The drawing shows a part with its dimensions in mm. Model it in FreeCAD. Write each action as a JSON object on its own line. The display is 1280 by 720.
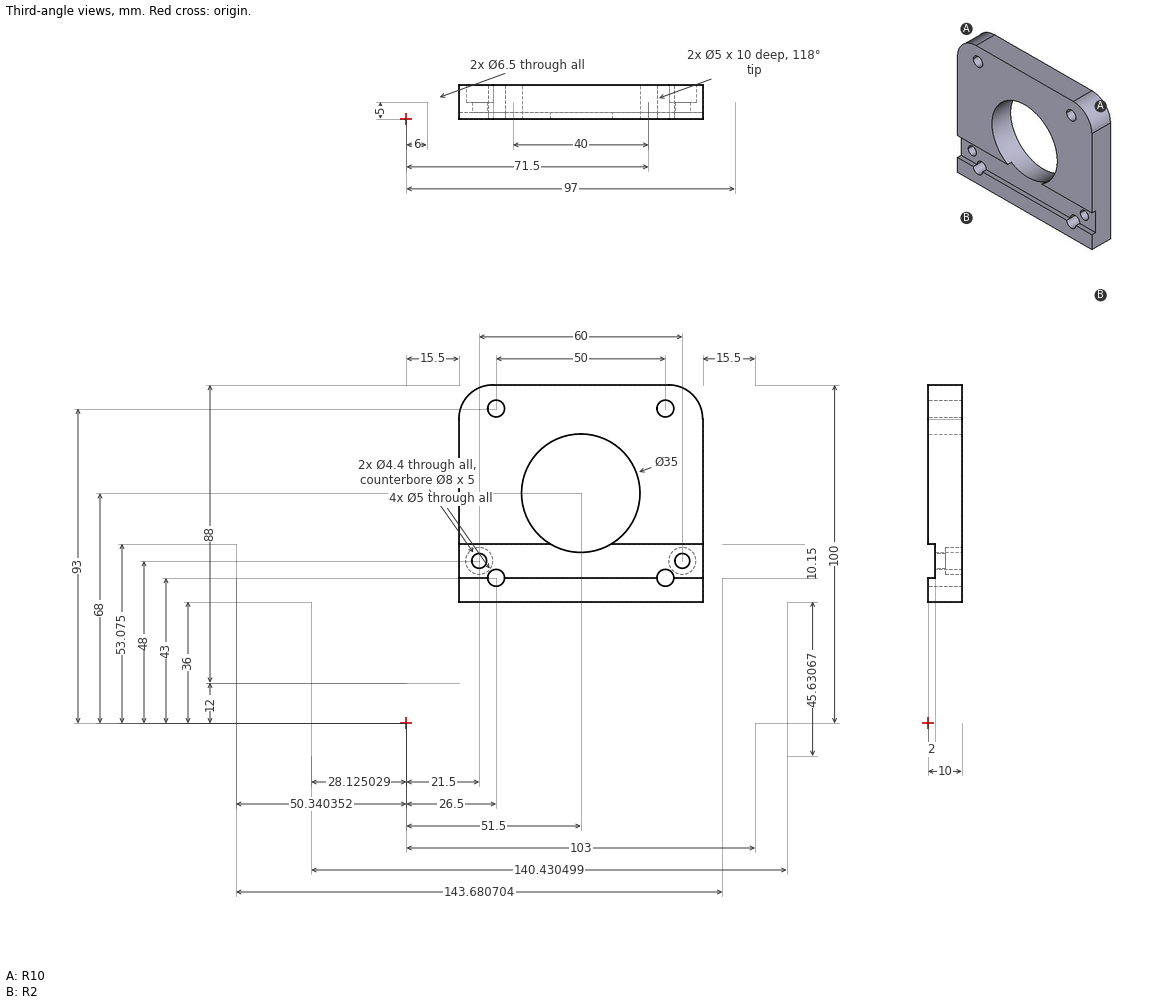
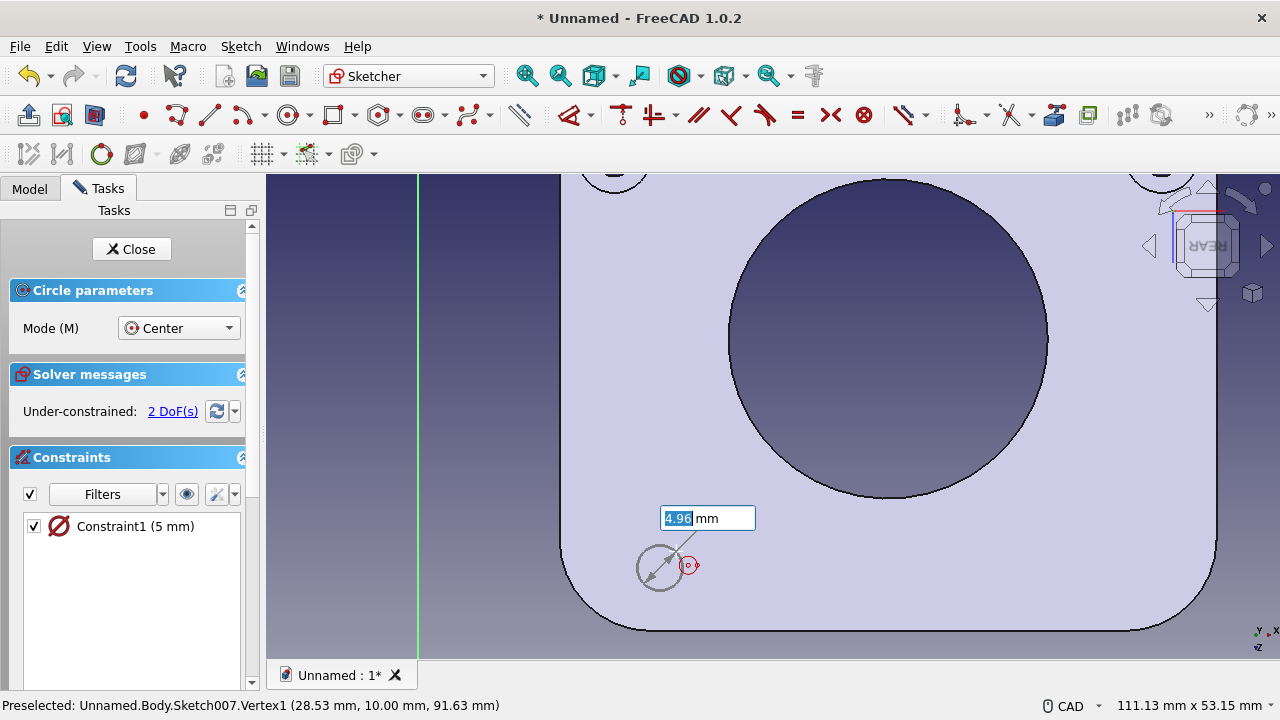
{"action": "type", "text": "5"}
{"action": "key", "text": "Return"}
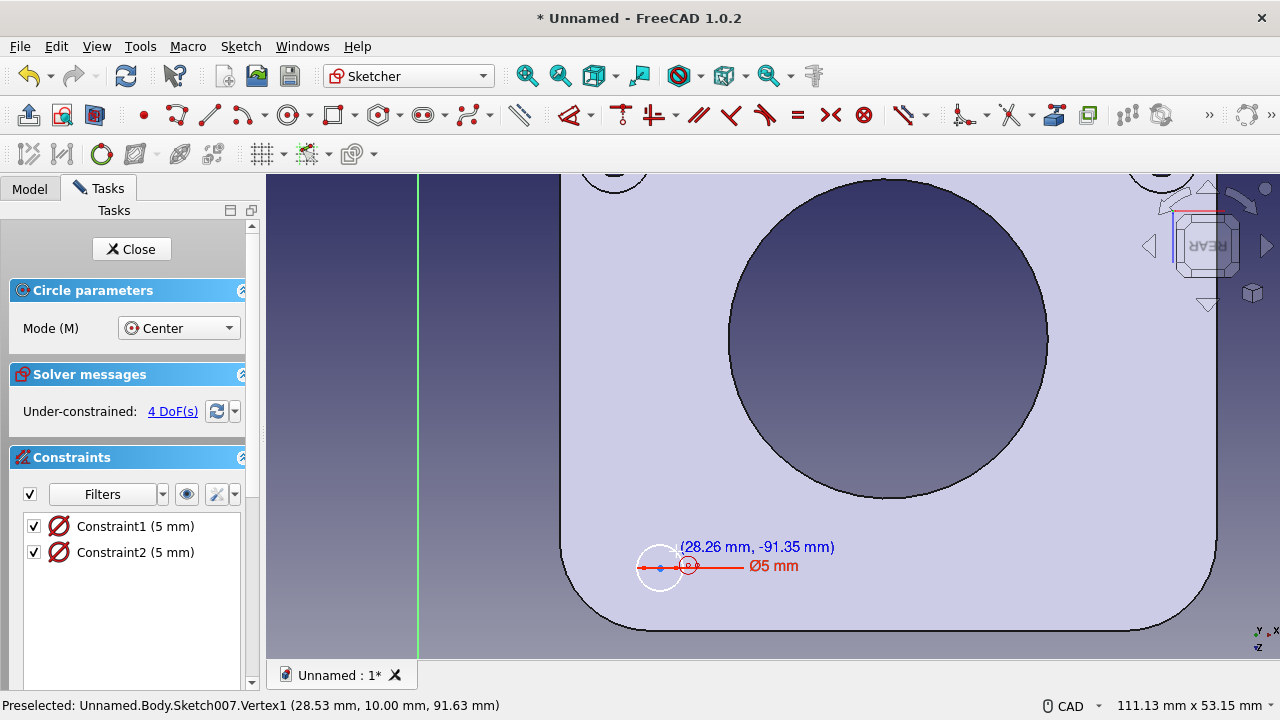
{"action": "scroll", "coordinate": [661, 569], "scroll_direction": "down", "scroll_amount": 5}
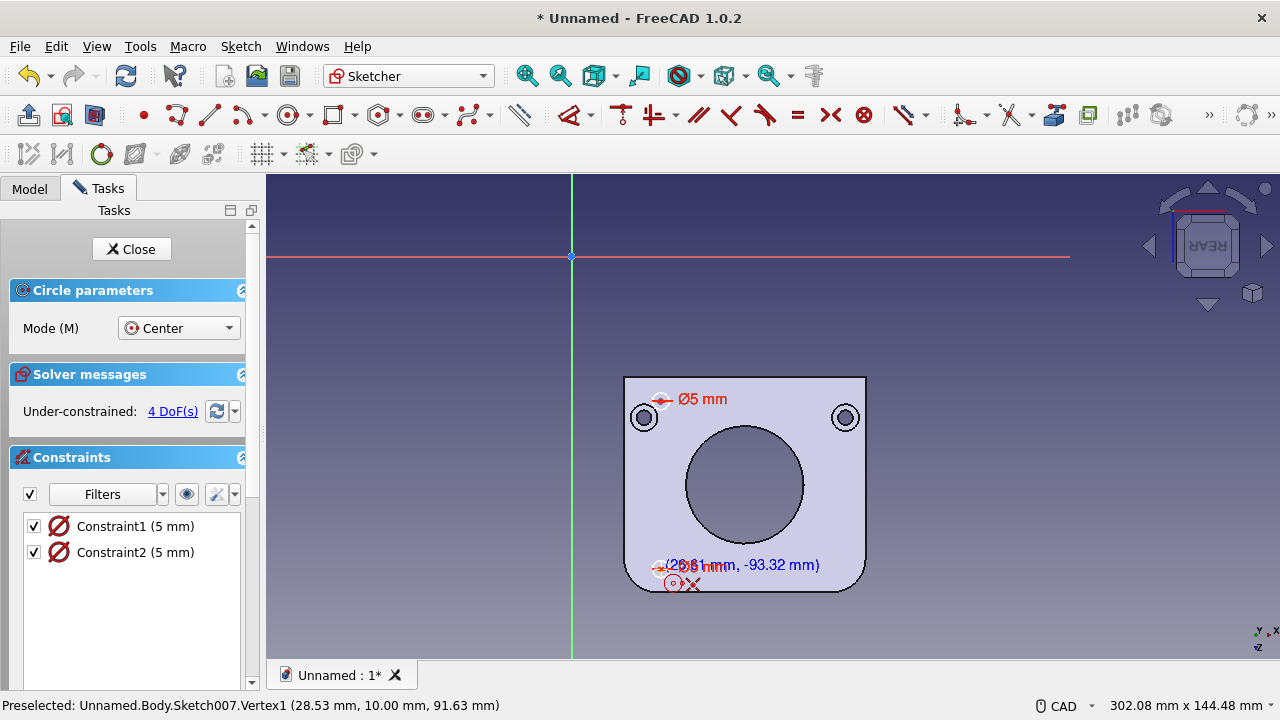
{"action": "scroll", "coordinate": [829, 569], "scroll_direction": "up", "scroll_amount": 5}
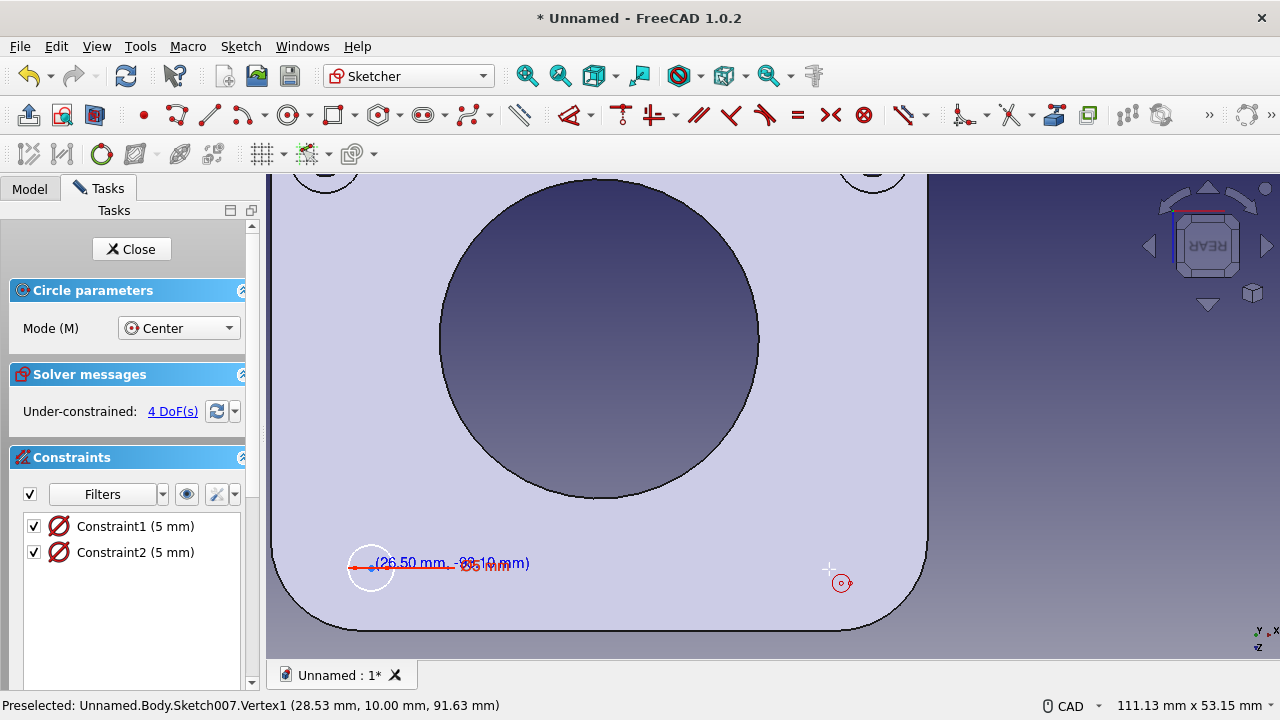
{"action": "left_click", "coordinate": [827, 567]}
{"action": "mouse_move", "coordinate": [843, 551]}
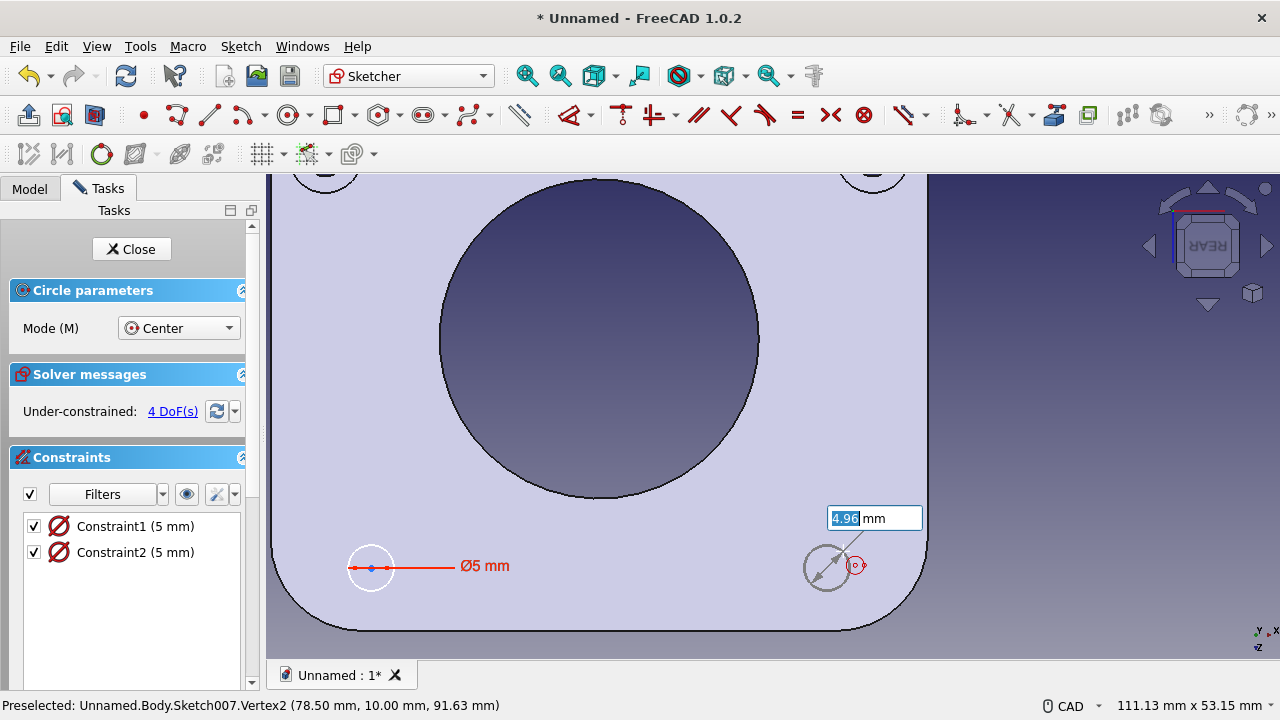
{"action": "type", "text": "5"}
{"action": "key", "text": "Return"}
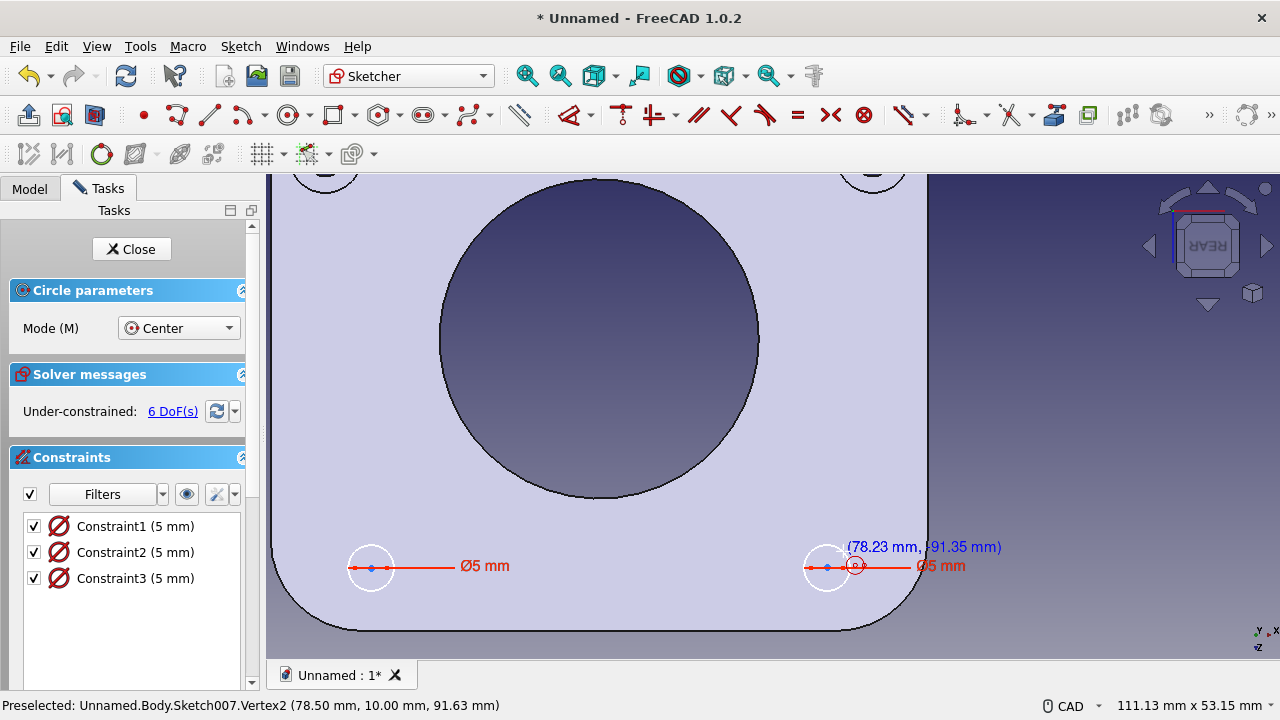
{"action": "scroll", "coordinate": [830, 569], "scroll_direction": "down", "scroll_amount": 5}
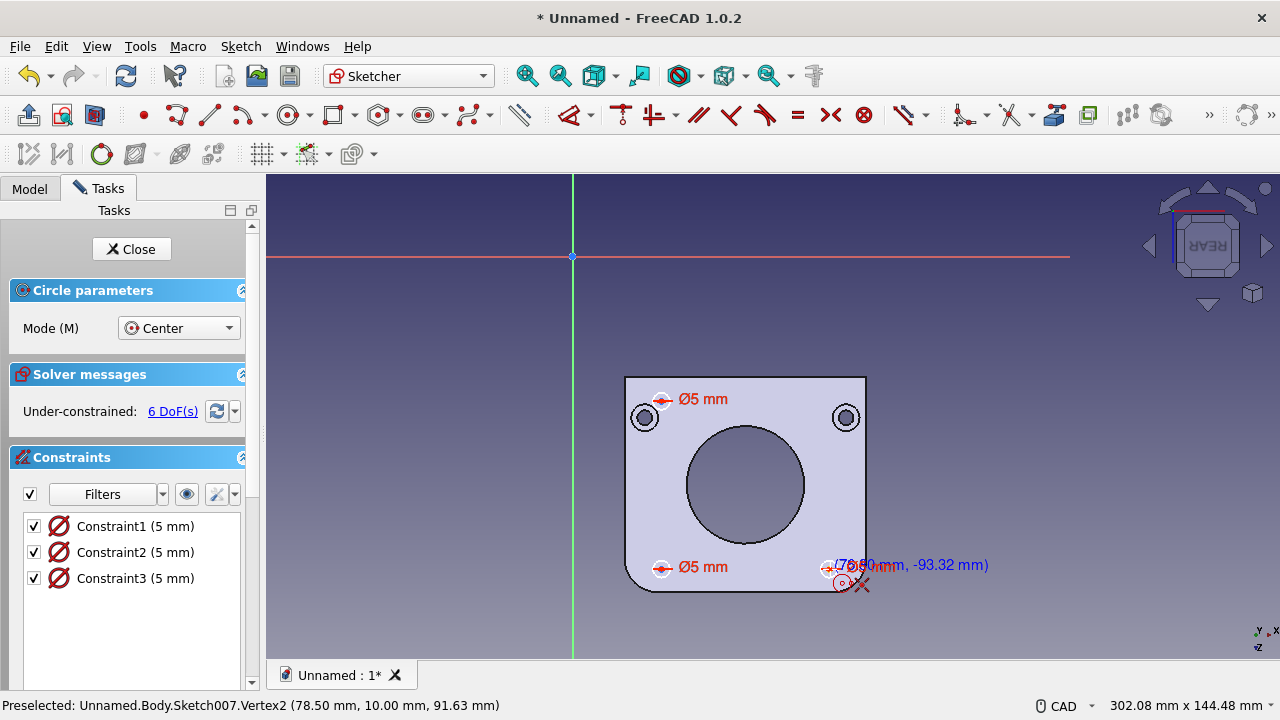
{"action": "scroll", "coordinate": [829, 401], "scroll_direction": "up", "scroll_amount": 5}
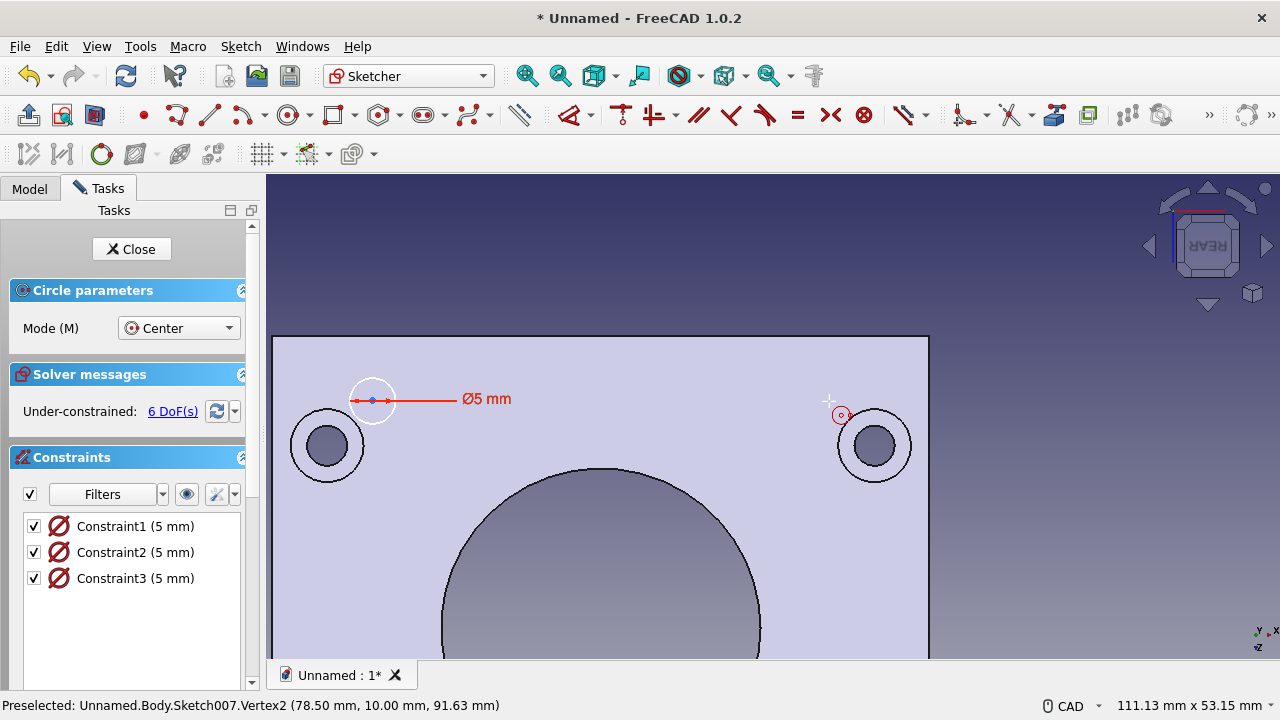
{"action": "left_click", "coordinate": [829, 400]}
{"action": "mouse_move", "coordinate": [845, 384]}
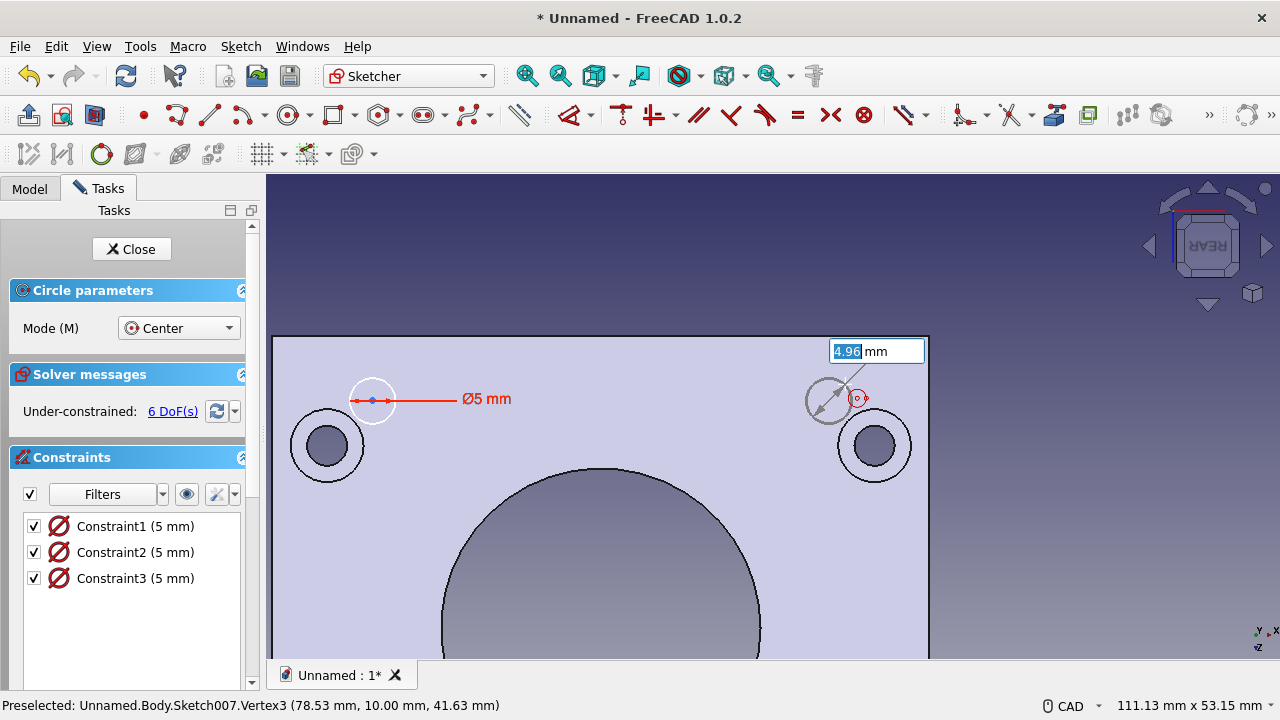
{"action": "type", "text": "5"}
{"action": "key", "text": "Return"}
{"action": "key", "text": "Escape"}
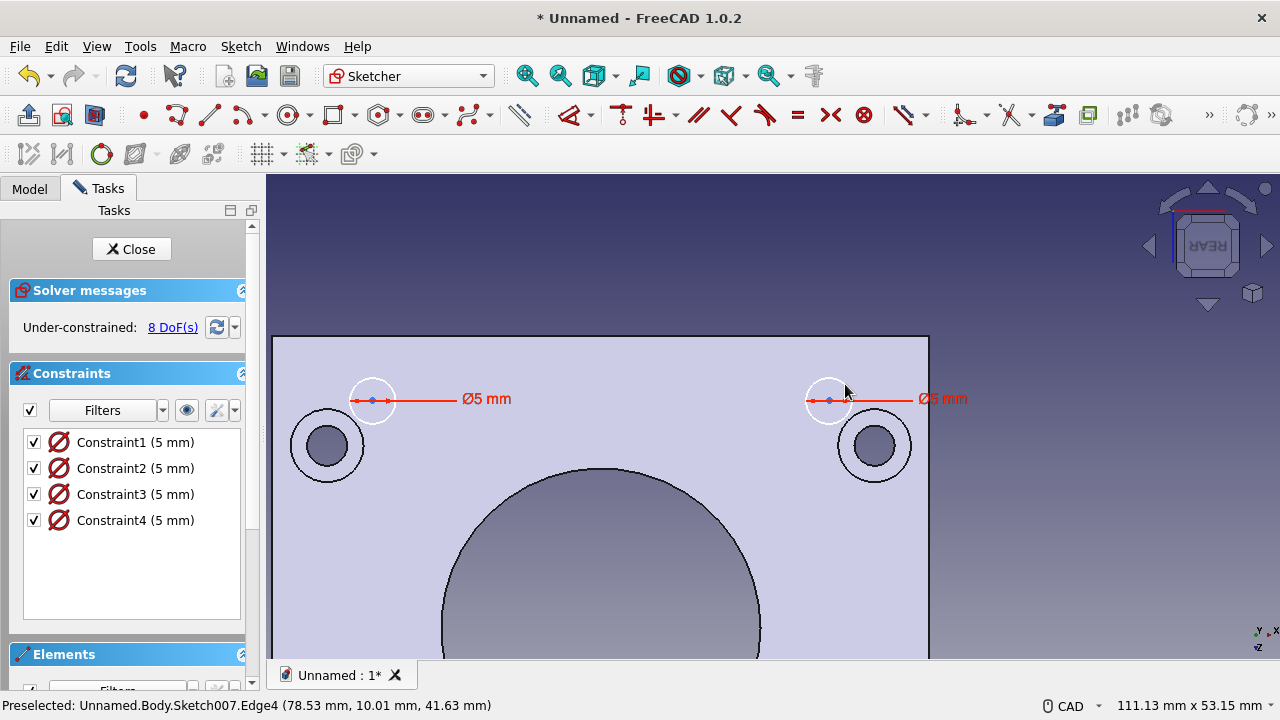
{"action": "left_click", "coordinate": [568, 116]}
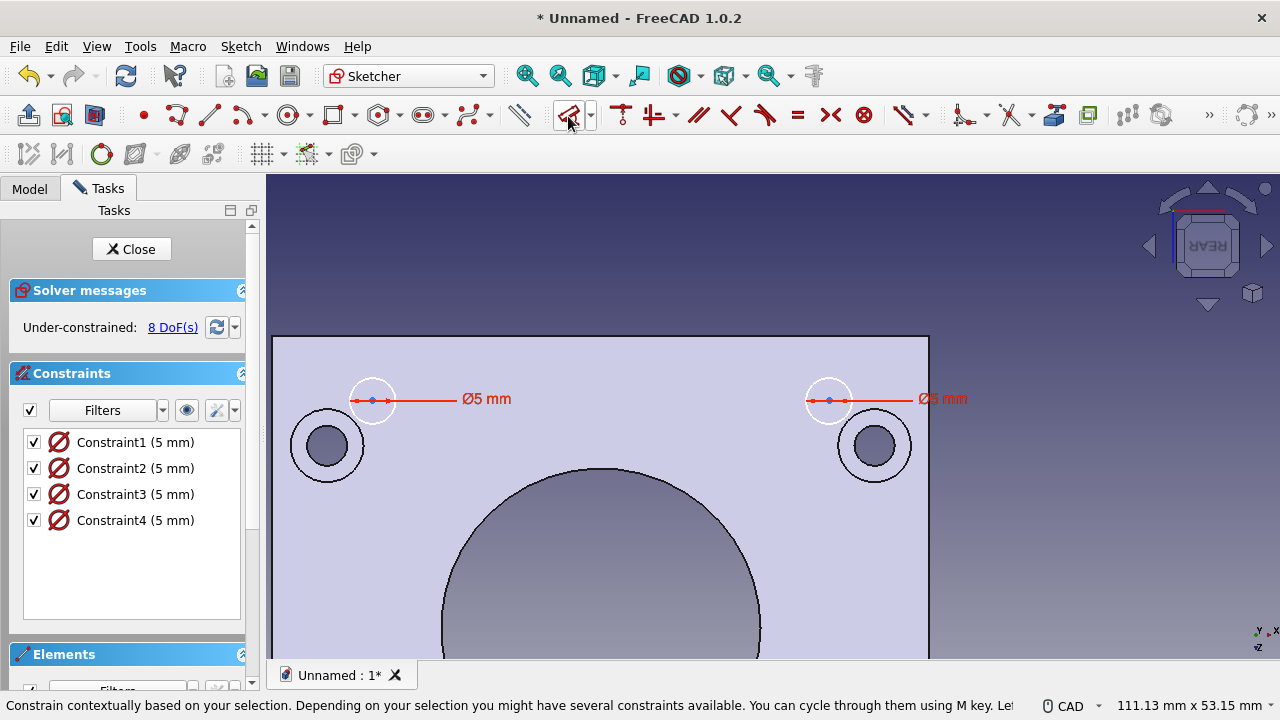
{"action": "left_click", "coordinate": [373, 401]}
{"action": "left_click", "coordinate": [407, 302]}